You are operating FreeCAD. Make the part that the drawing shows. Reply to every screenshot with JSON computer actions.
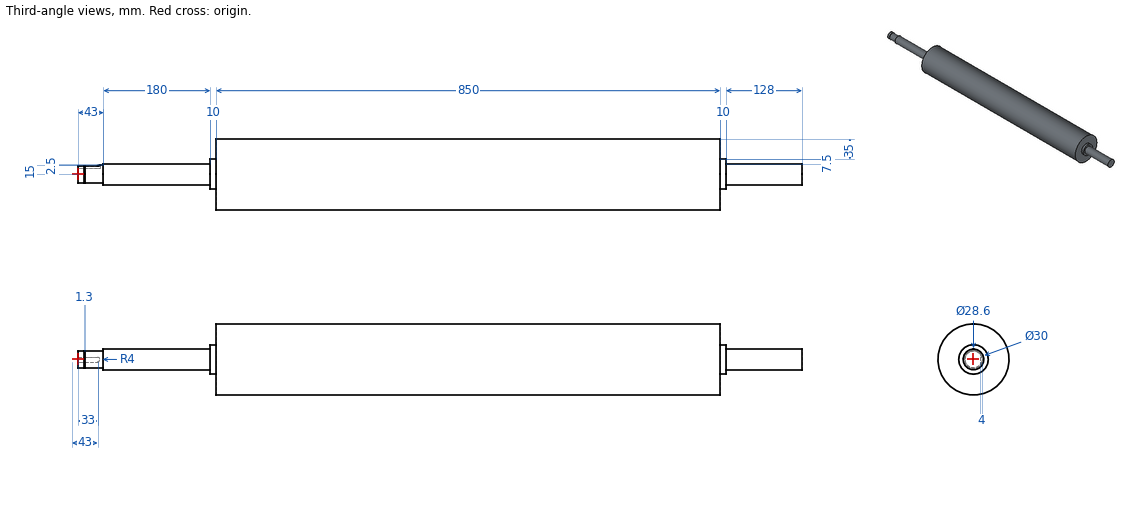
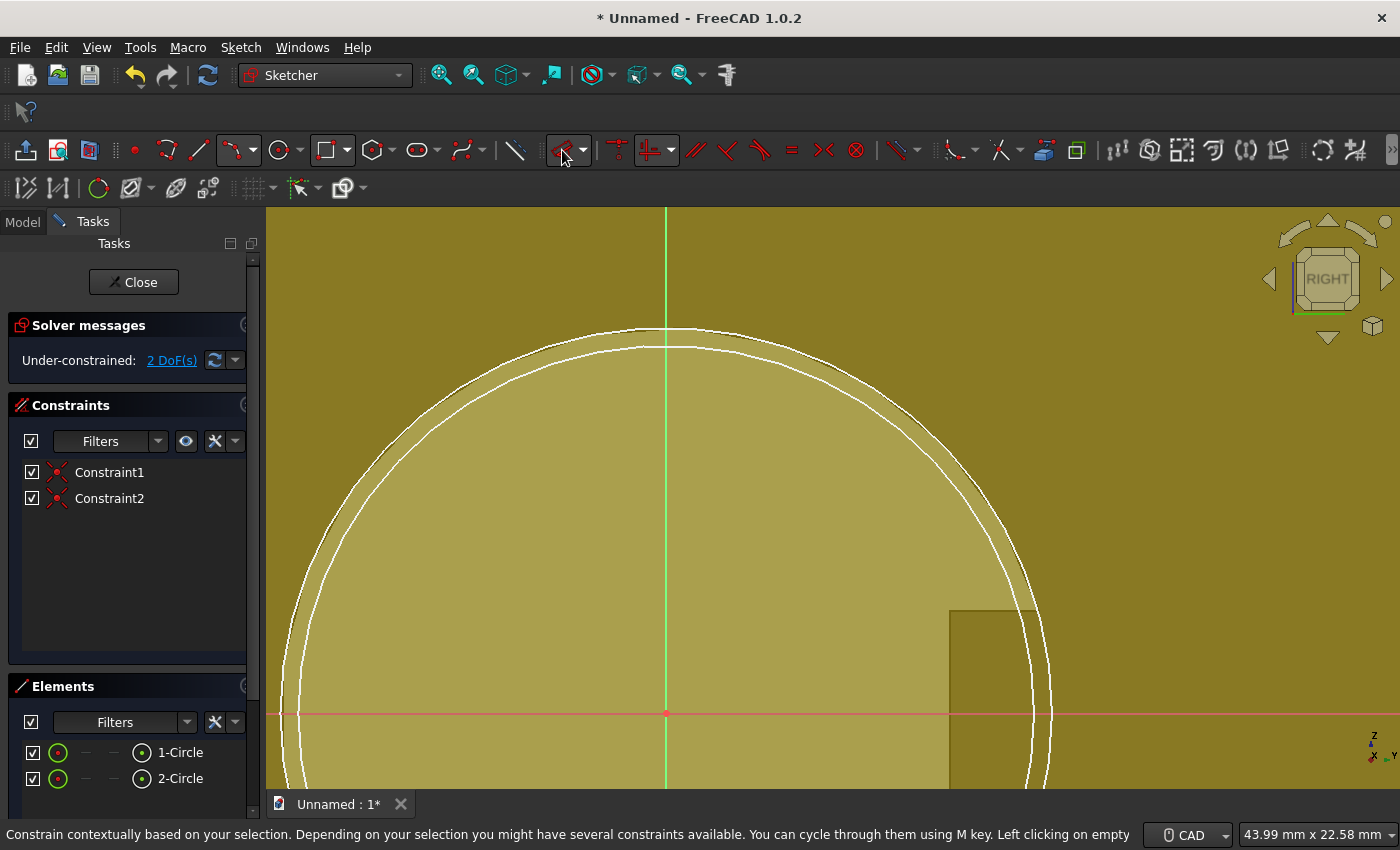
{"action": "left_click", "coordinate": [938, 440]}
{"action": "left_click", "coordinate": [961, 417]}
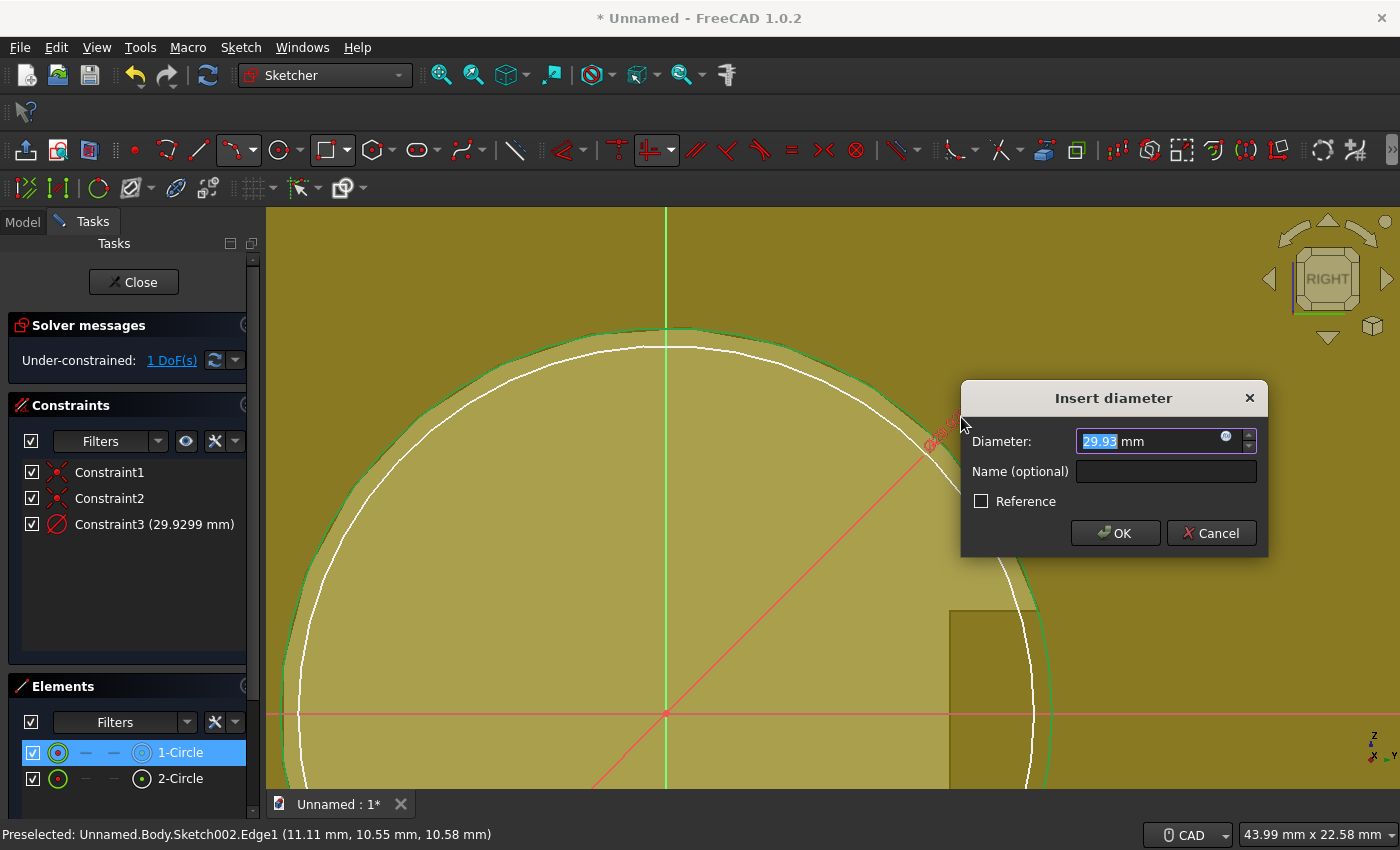
{"action": "type", "text": "30"}
{"action": "key", "text": "Return"}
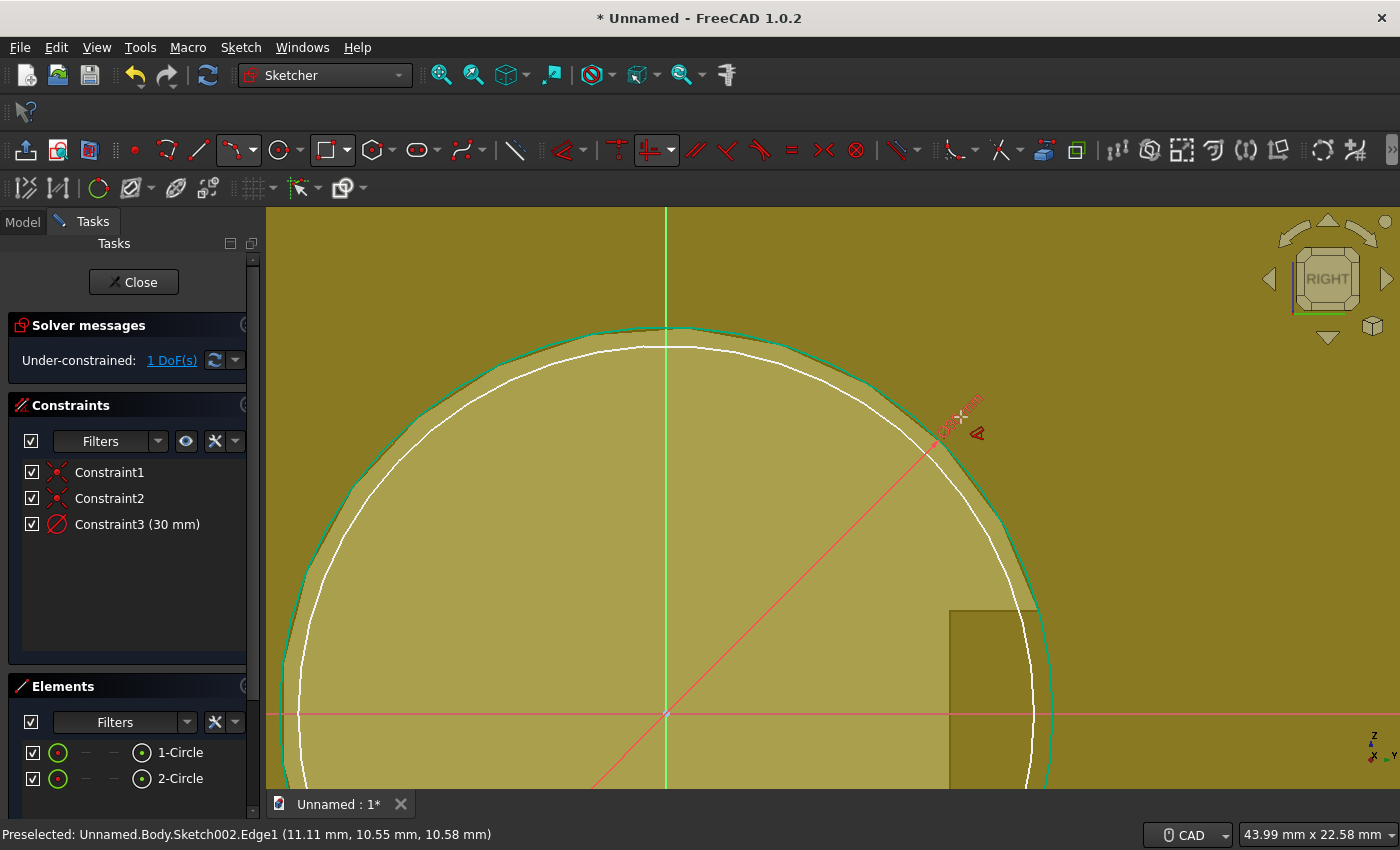
{"action": "left_click", "coordinate": [926, 453]}
{"action": "left_click", "coordinate": [1050, 600]}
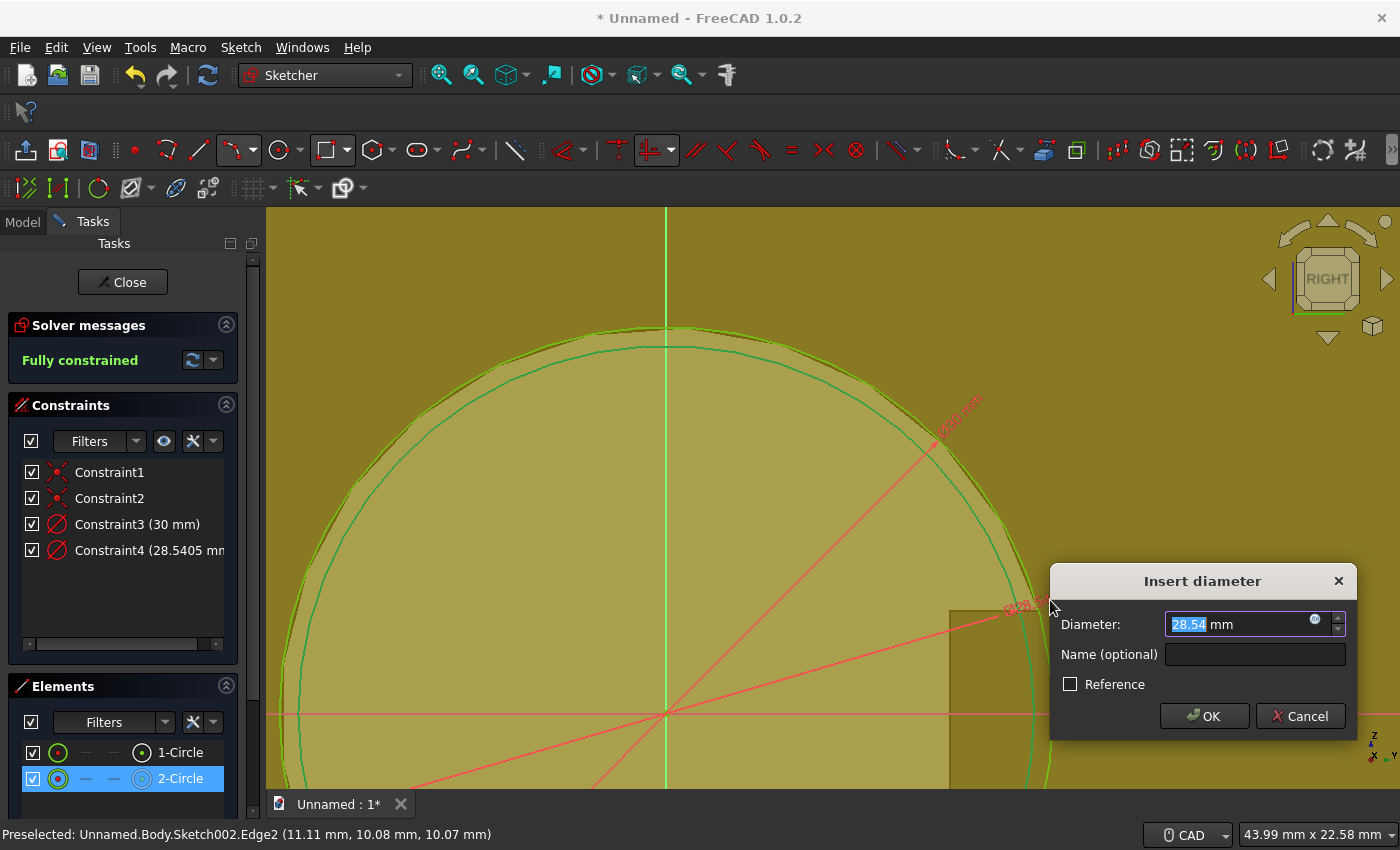
{"action": "type", "text": "28.6"}
{"action": "key", "text": "Return"}
{"action": "key", "text": "Escape"}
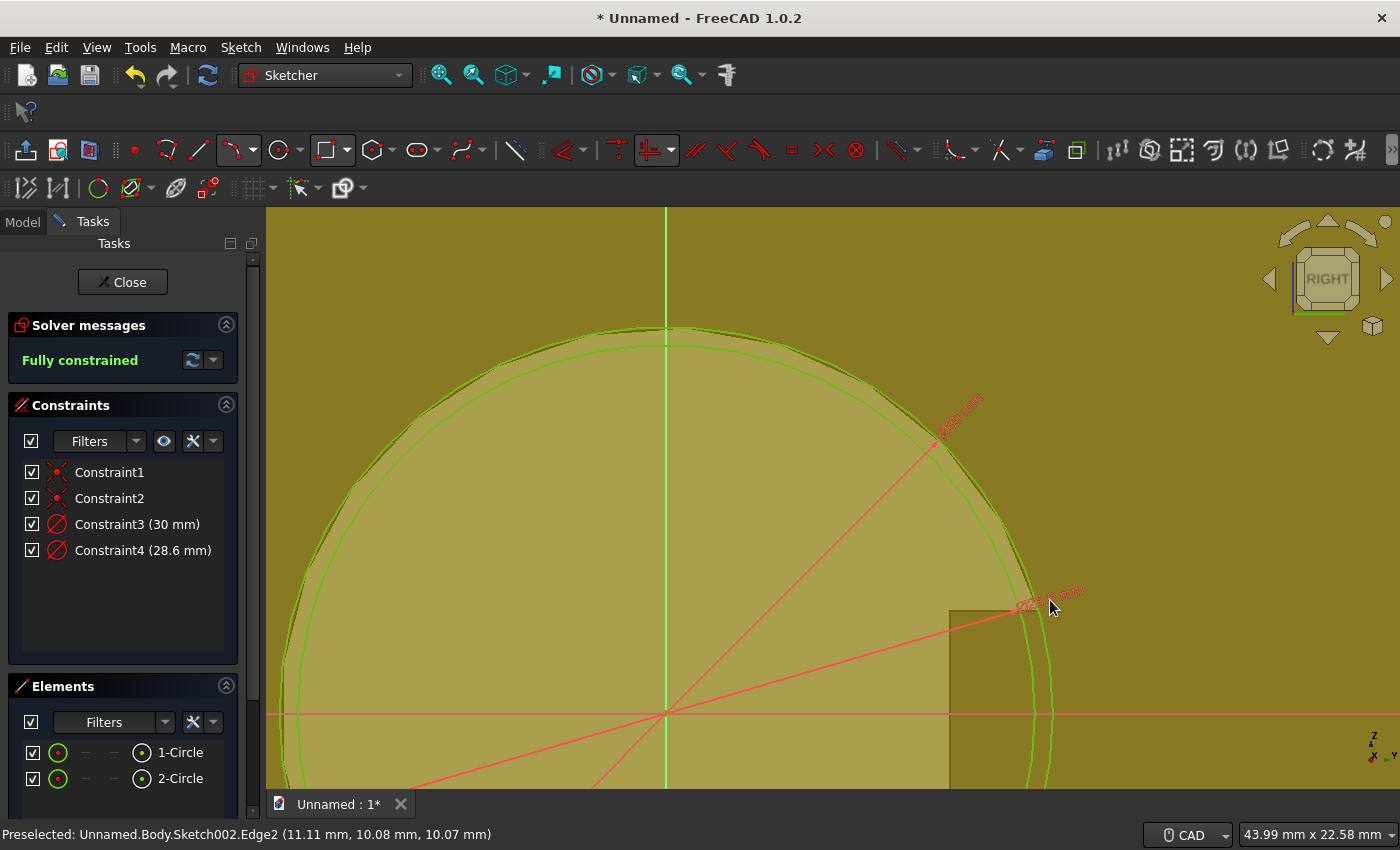
{"action": "left_click", "coordinate": [123, 282]}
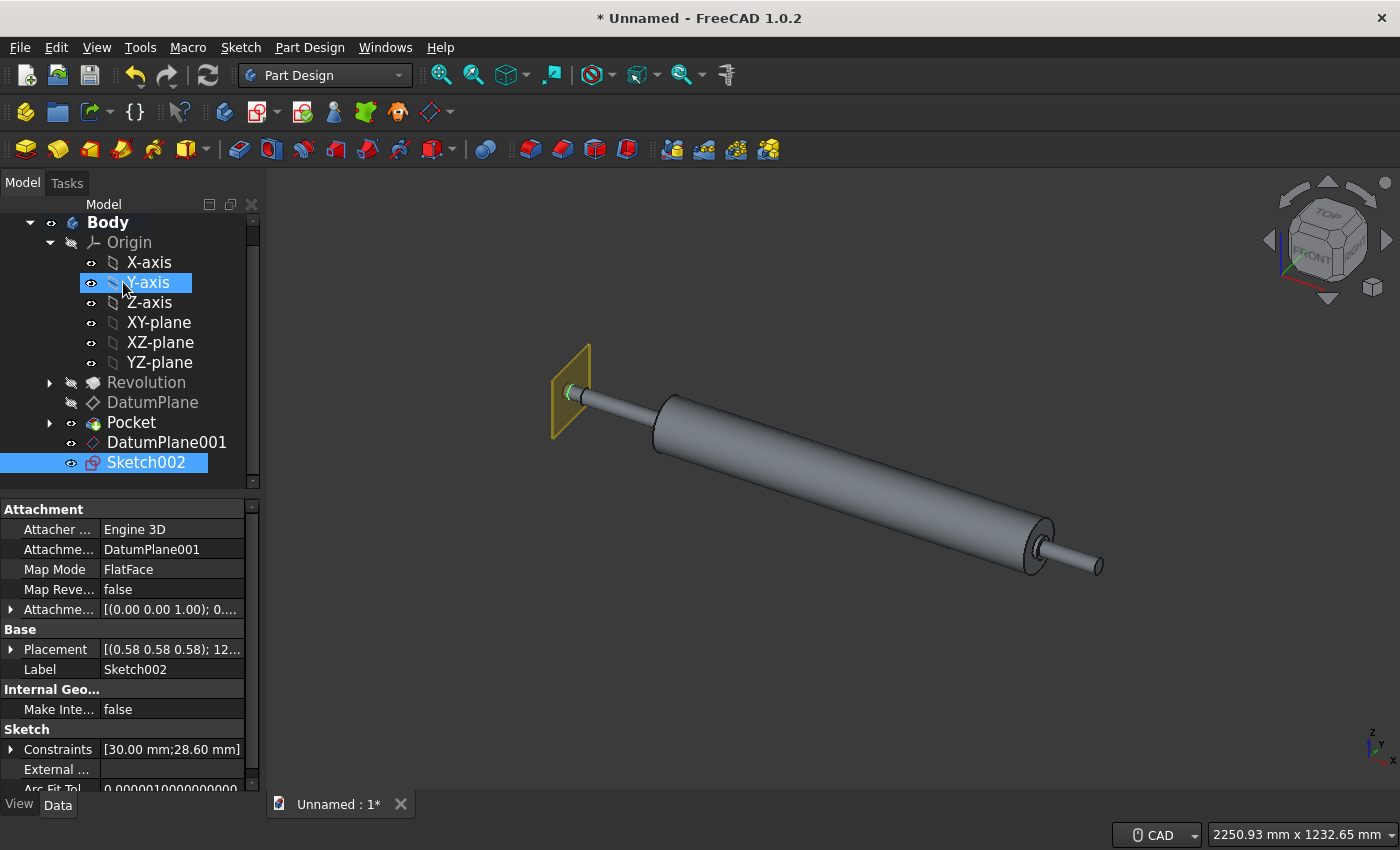
{"action": "left_click", "coordinate": [240, 150]}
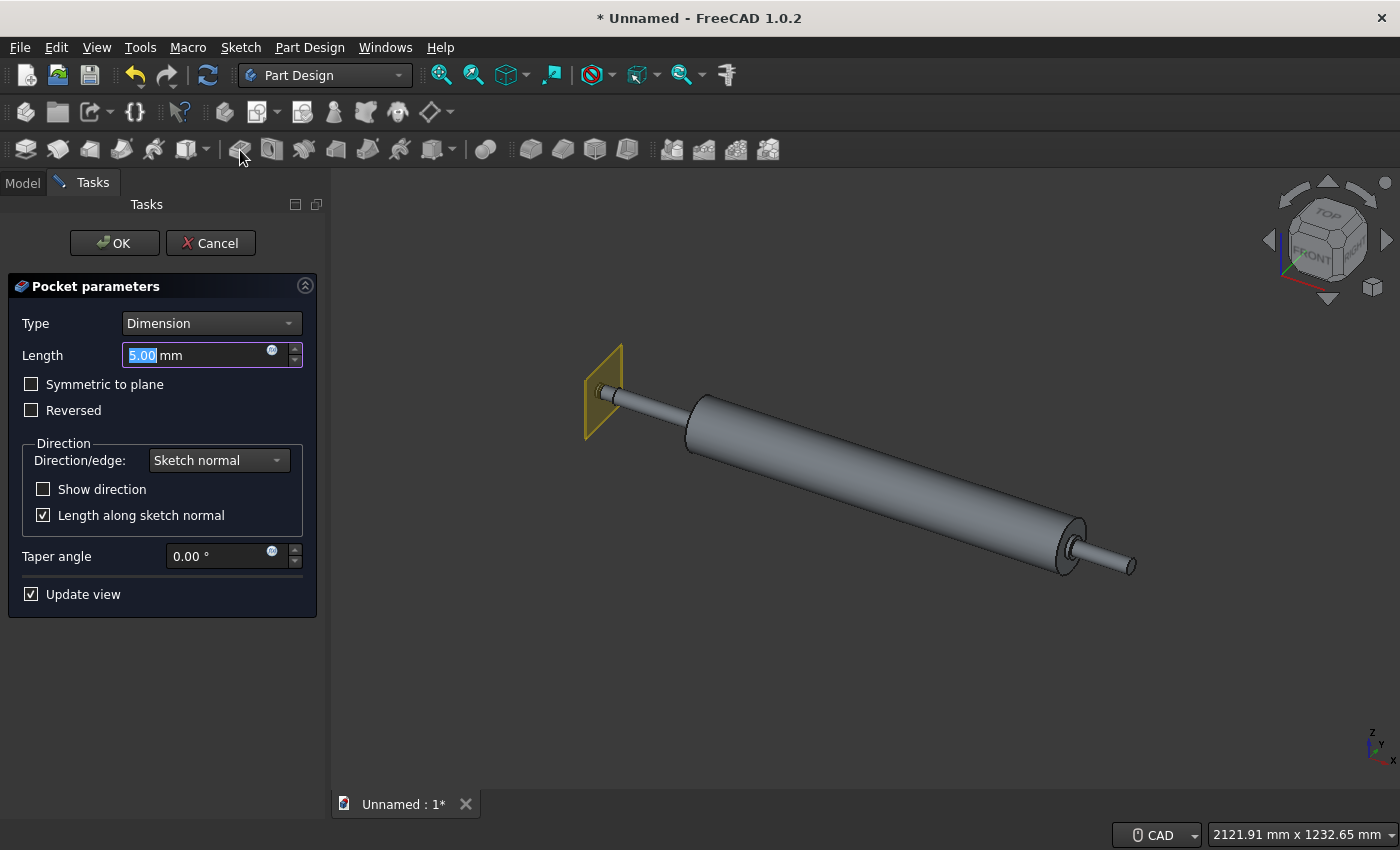
{"action": "type", "text": "1.3"}
{"action": "key", "text": "Tab"}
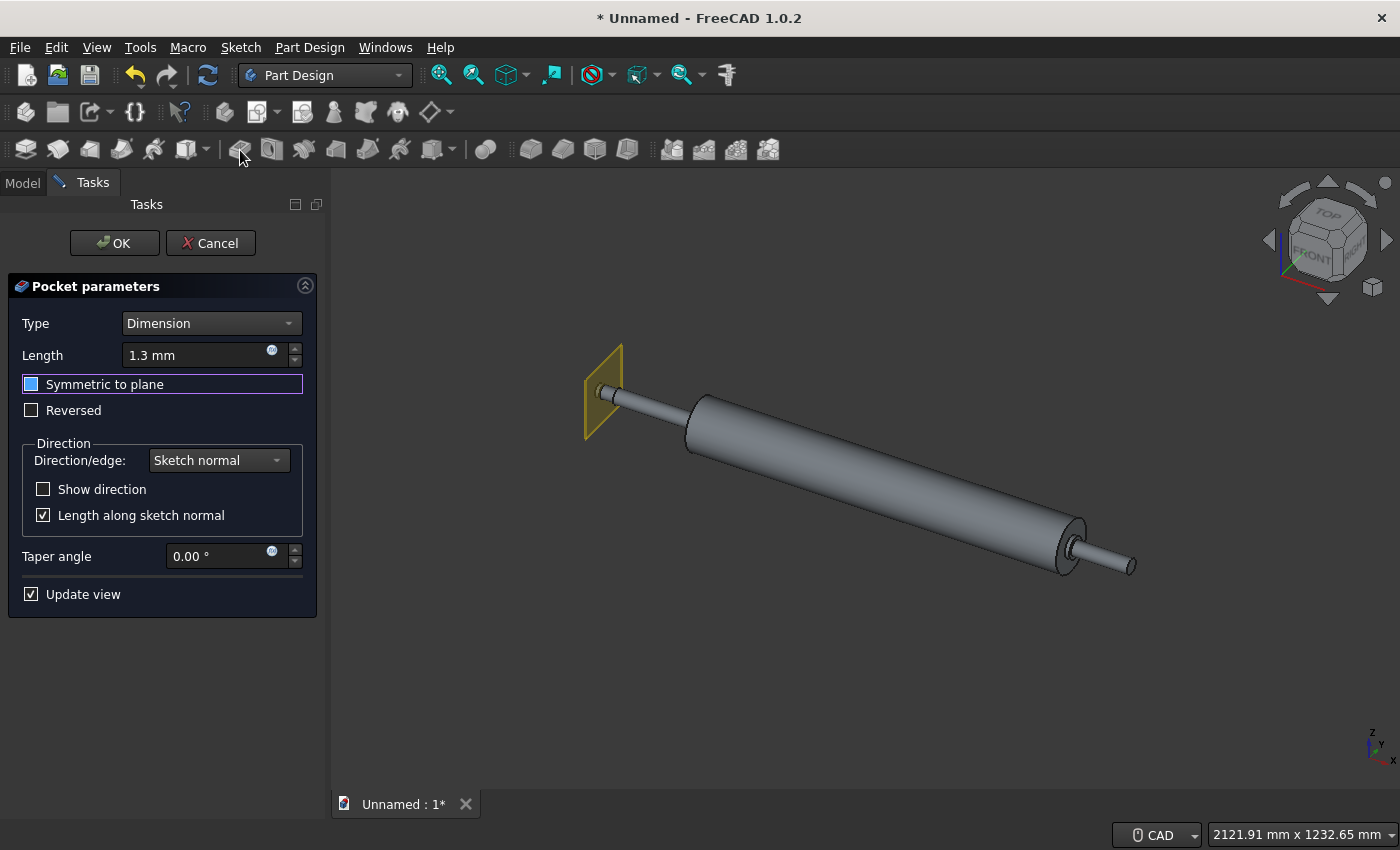
{"action": "left_click", "coordinate": [115, 243]}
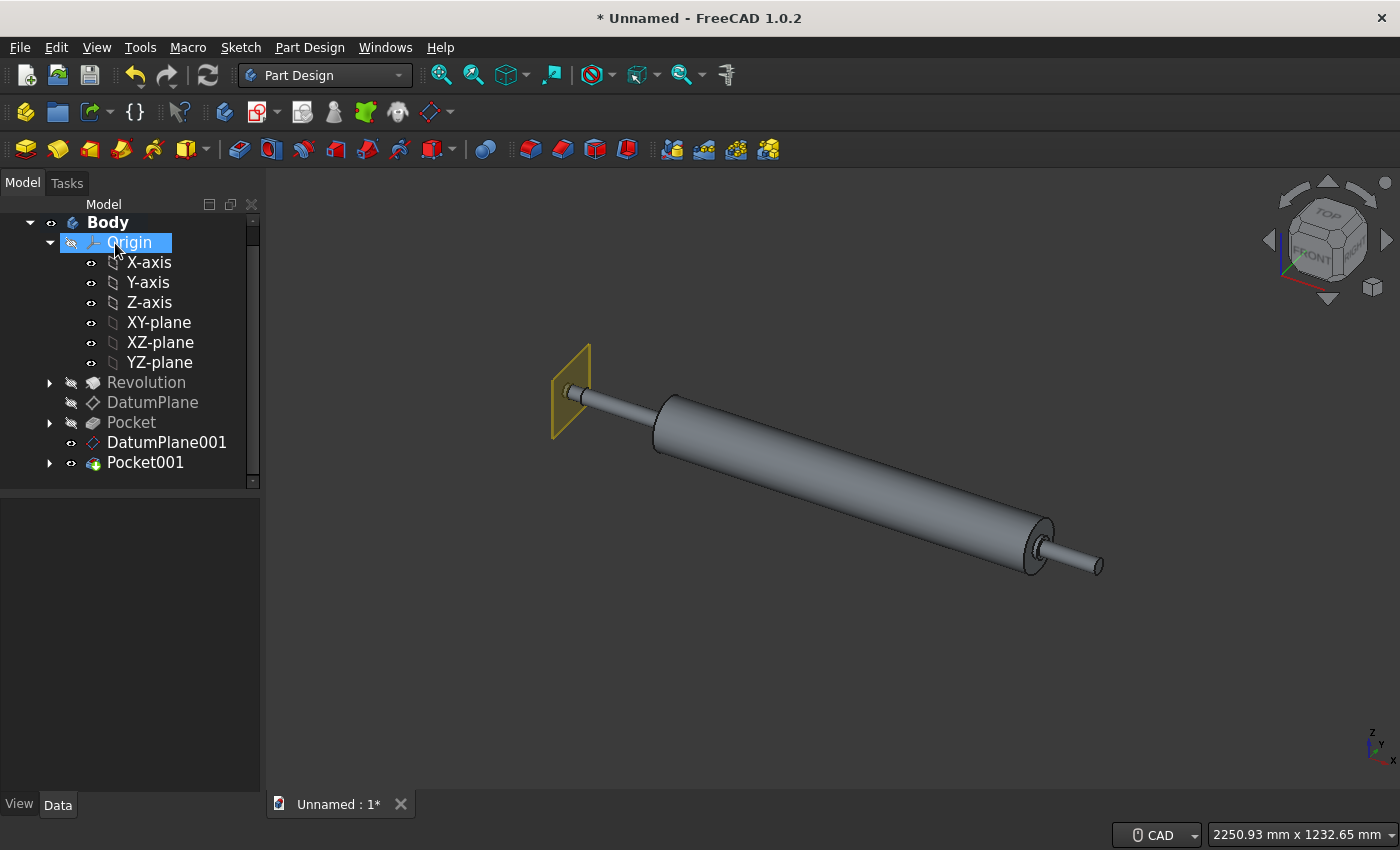
{"action": "left_click", "coordinate": [116, 443]}
{"action": "key", "text": "space"}